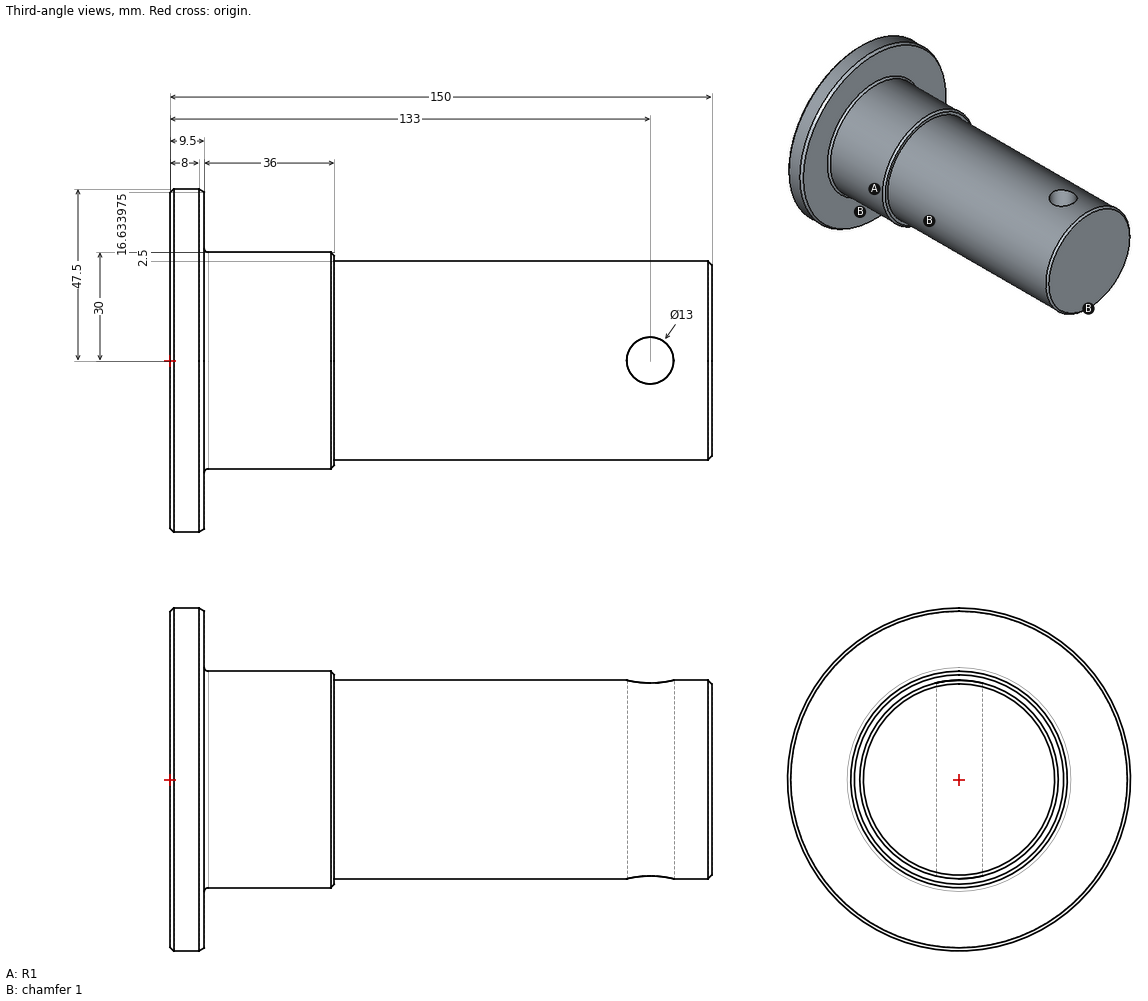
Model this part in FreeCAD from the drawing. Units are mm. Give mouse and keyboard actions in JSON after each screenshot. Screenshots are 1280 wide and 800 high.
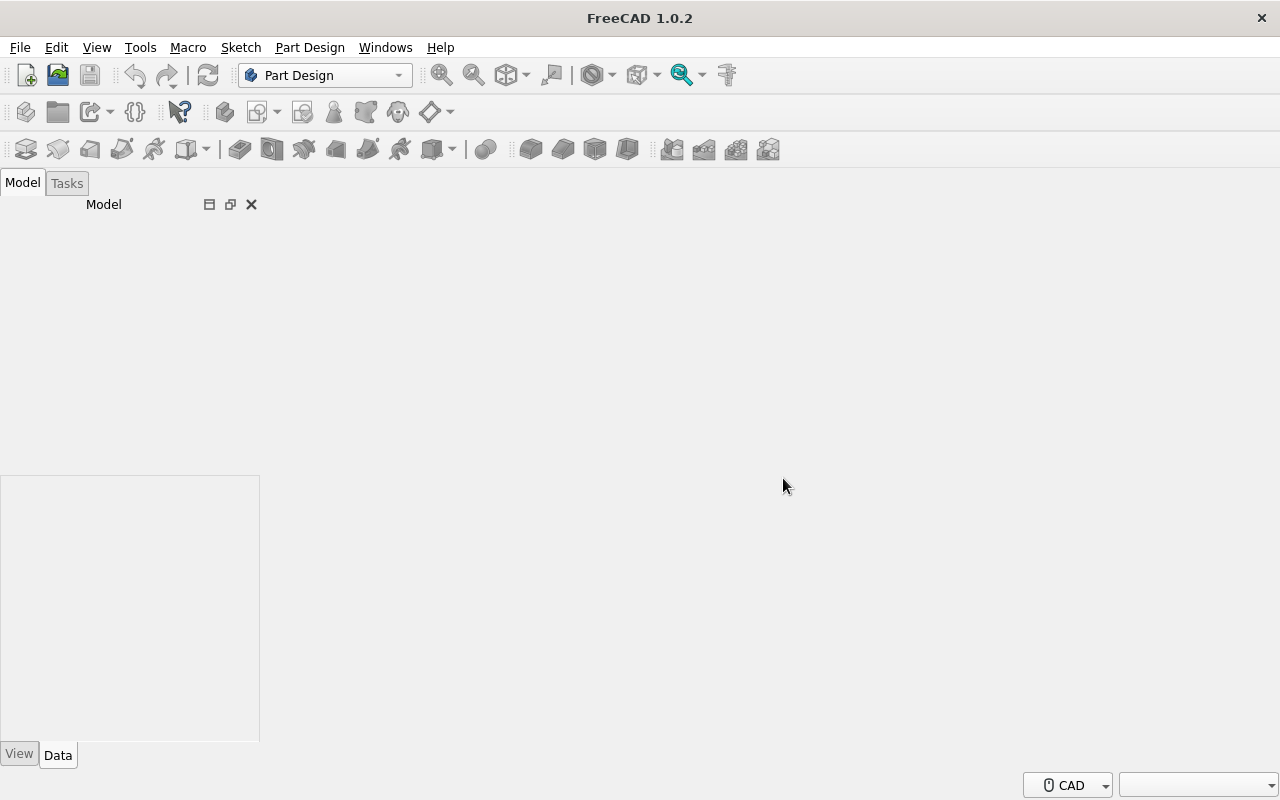
{"action": "key", "text": "ctrl+n"}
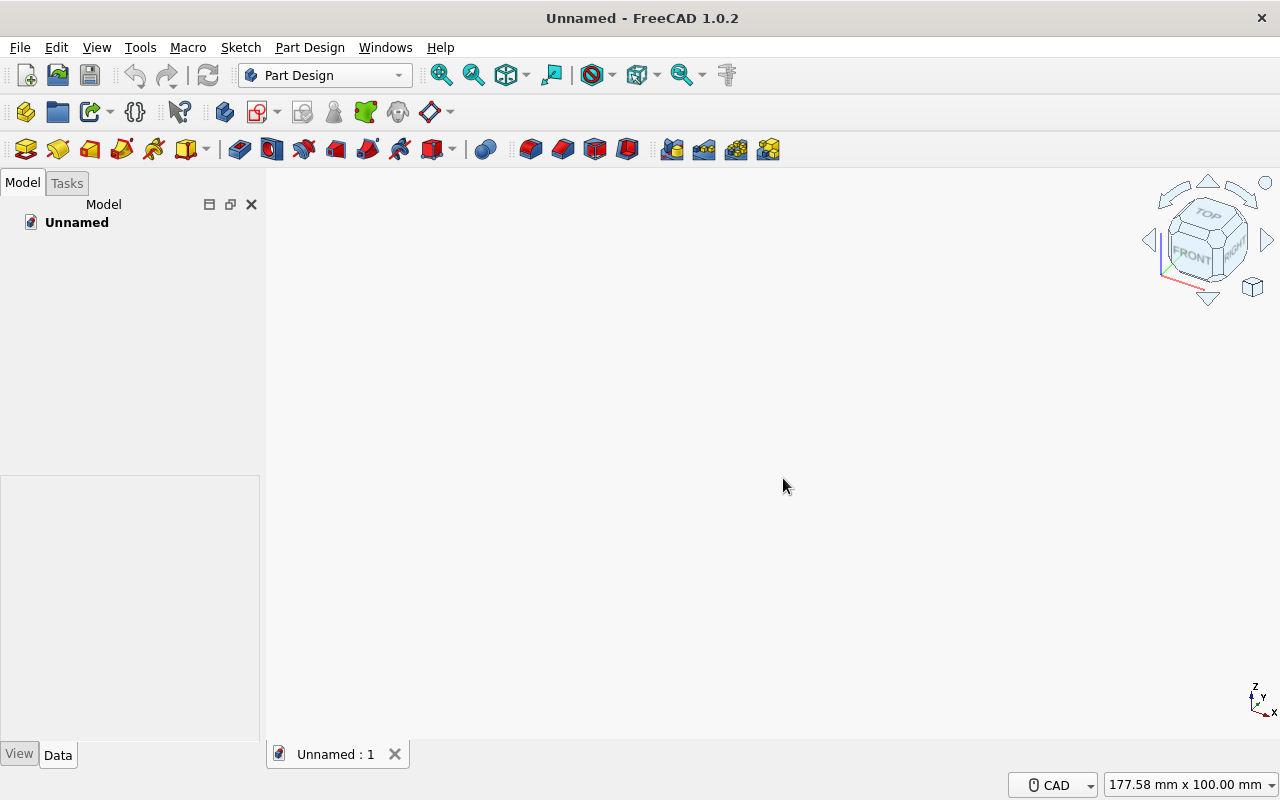
{"action": "left_click", "coordinate": [258, 112]}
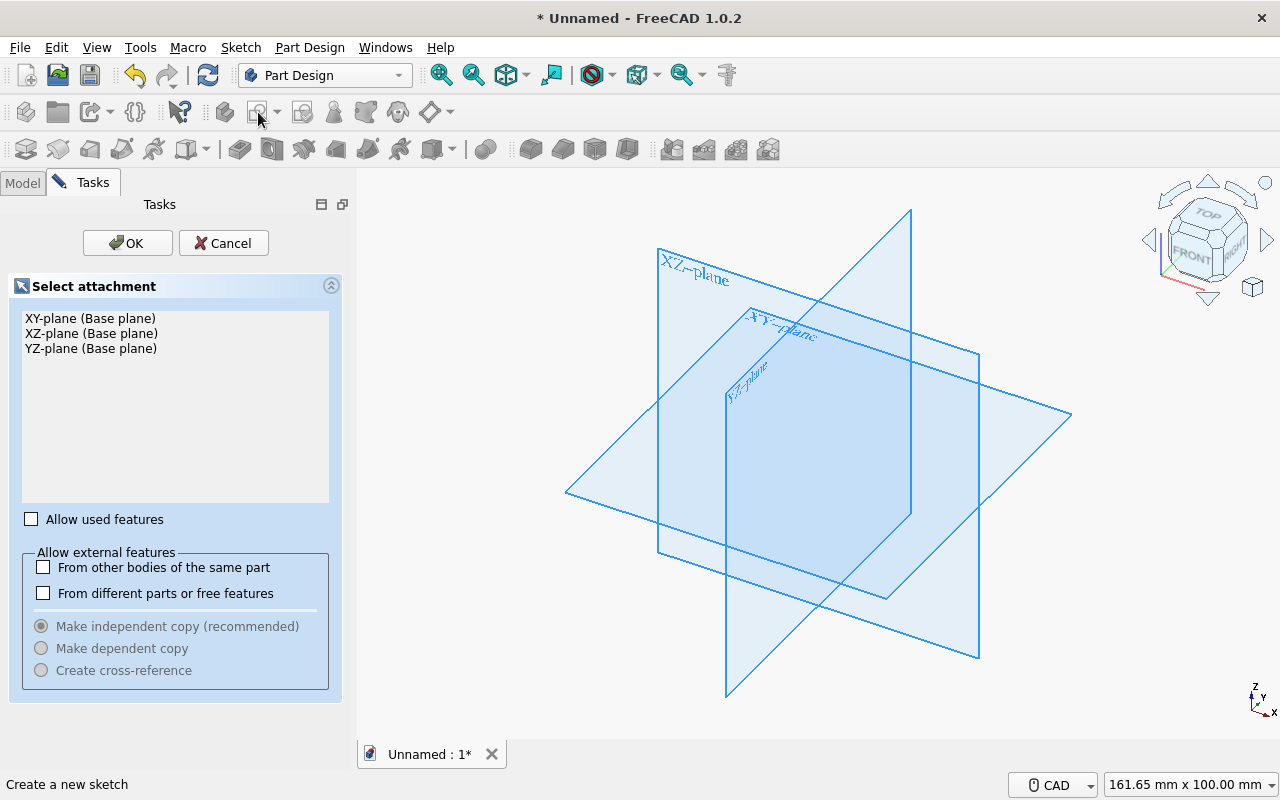
{"action": "left_click", "coordinate": [82, 318]}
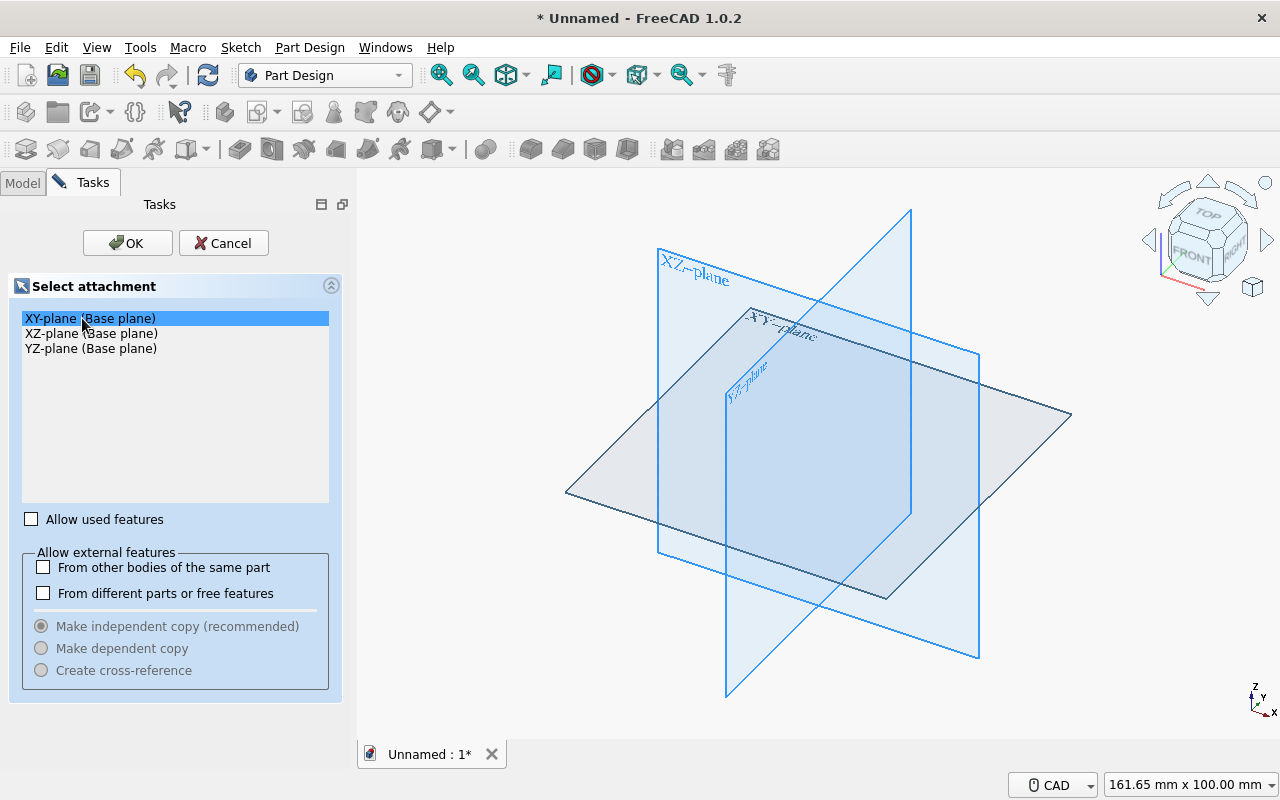
{"action": "left_click", "coordinate": [128, 243]}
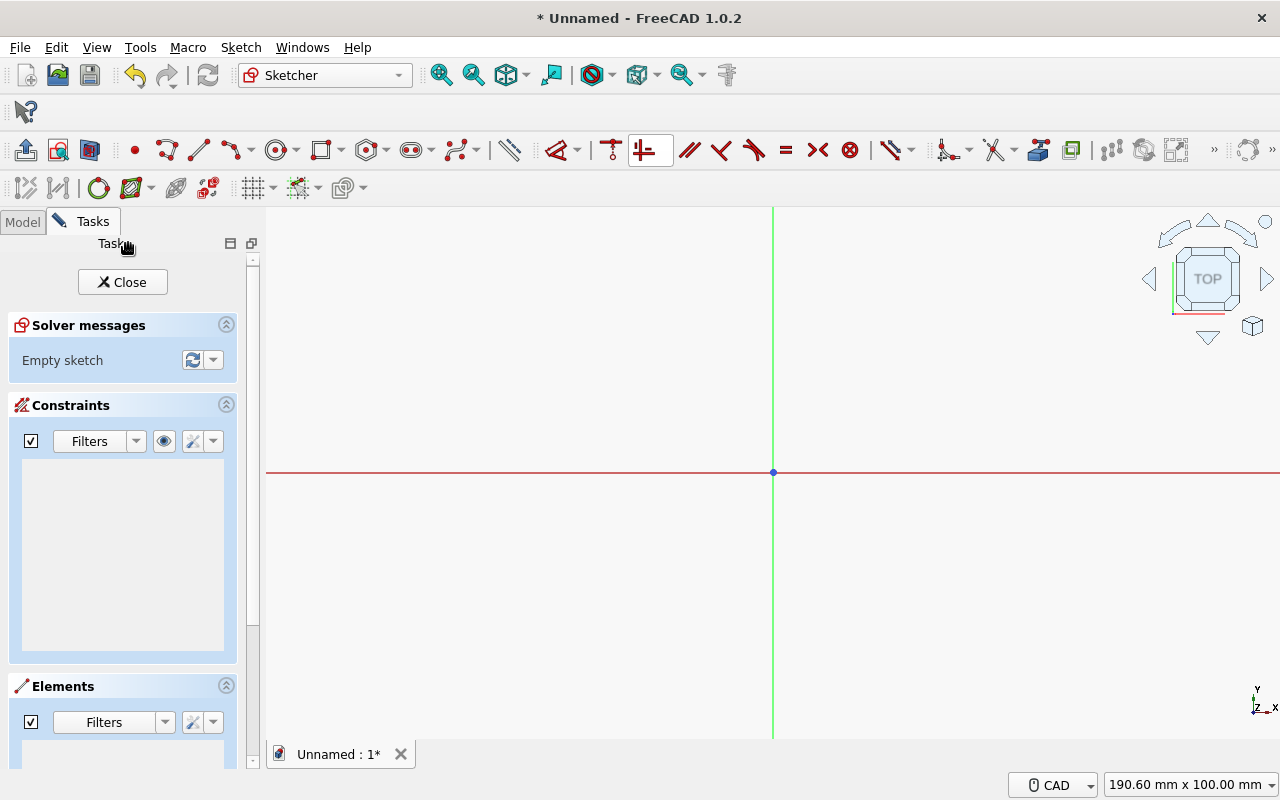
{"action": "scroll", "coordinate": [294, 627], "scroll_direction": "down", "scroll_amount": 3}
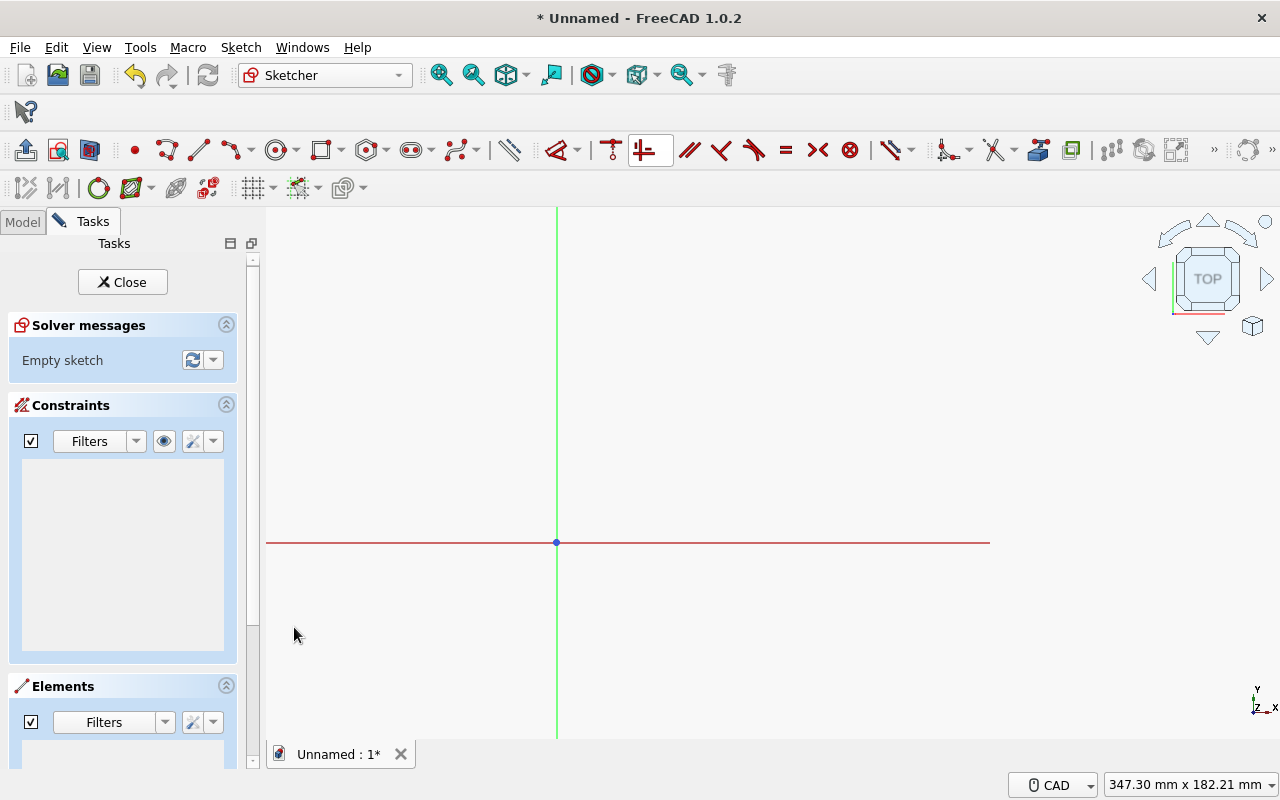
{"action": "key", "text": "g m"}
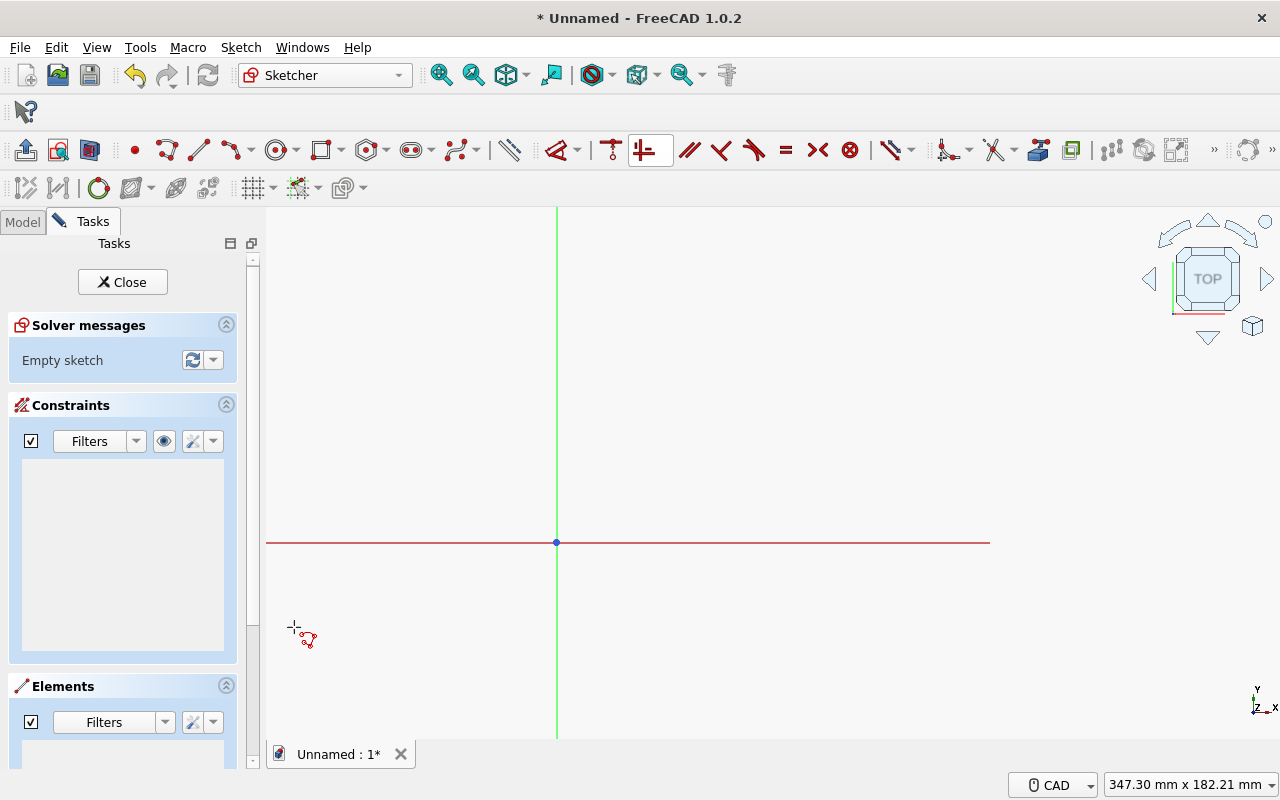
{"action": "left_click", "coordinate": [557, 543]}
{"action": "left_click", "coordinate": [995, 534]}
{"action": "left_click", "coordinate": [995, 463]}
{"action": "left_click", "coordinate": [690, 463]}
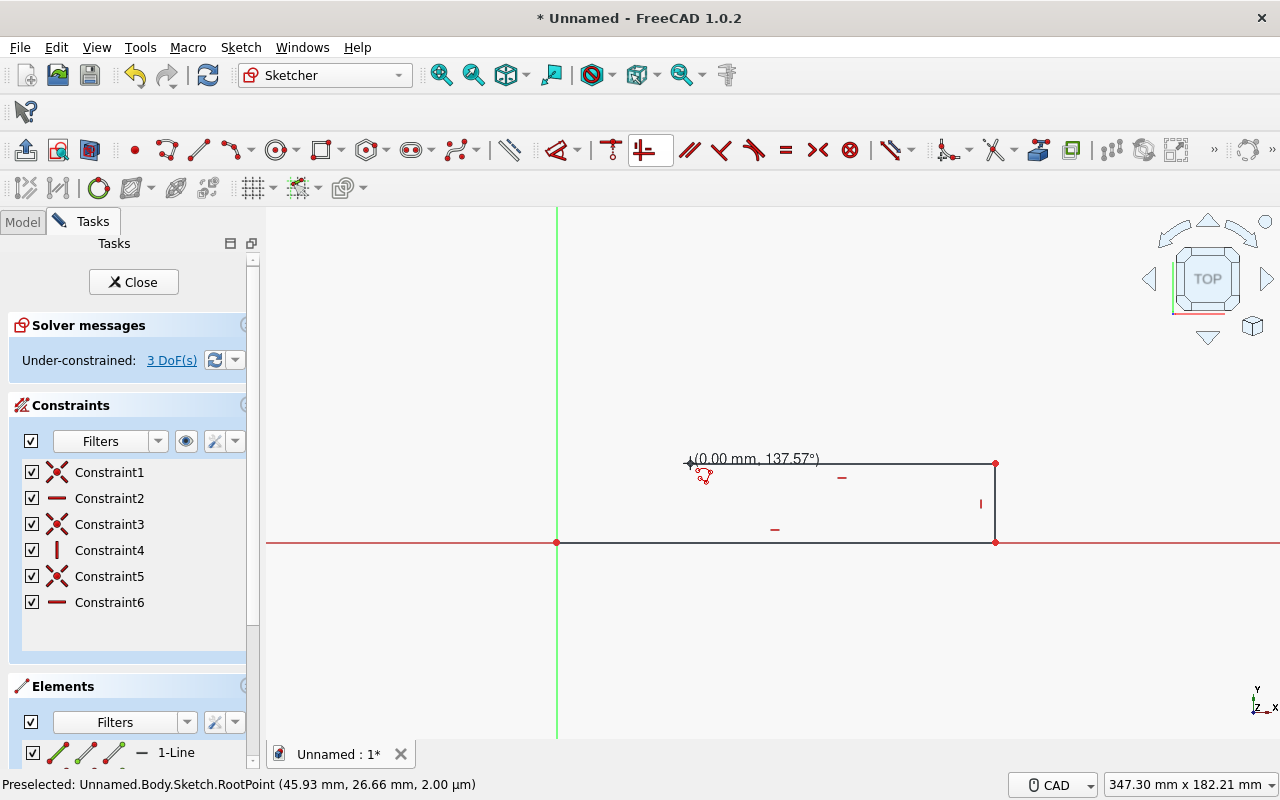
{"action": "scroll", "coordinate": [690, 455], "scroll_direction": "up", "scroll_amount": 4}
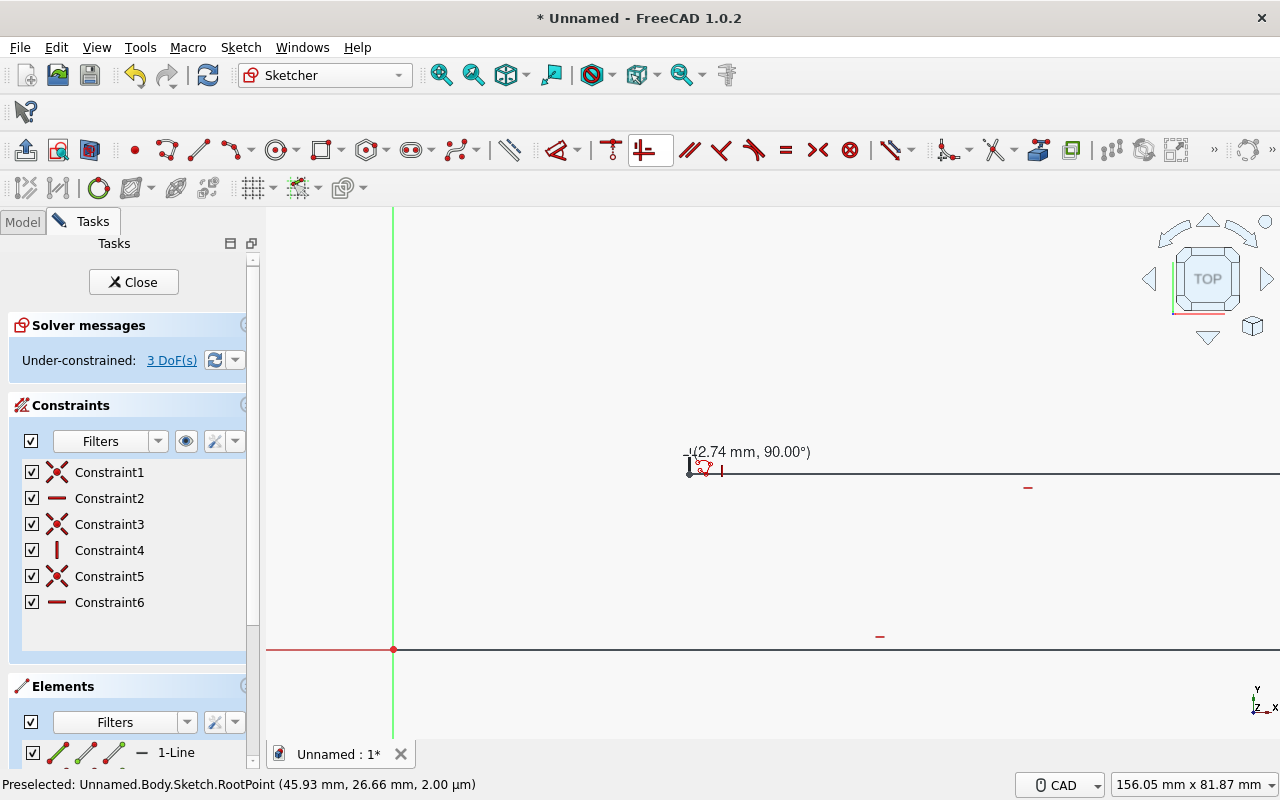
{"action": "left_click", "coordinate": [689, 455]}
{"action": "left_click", "coordinate": [455, 455]}
{"action": "left_click", "coordinate": [455, 347]}